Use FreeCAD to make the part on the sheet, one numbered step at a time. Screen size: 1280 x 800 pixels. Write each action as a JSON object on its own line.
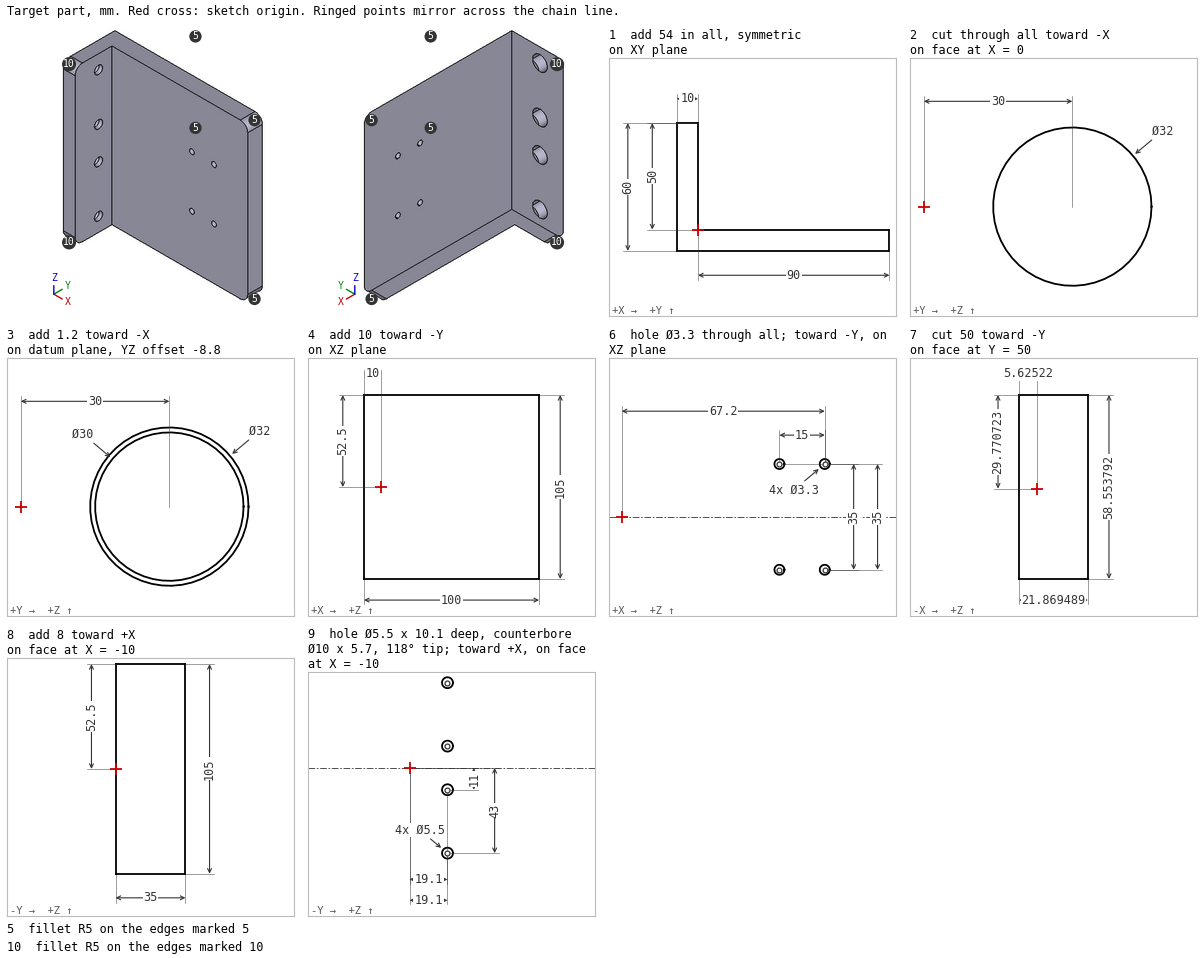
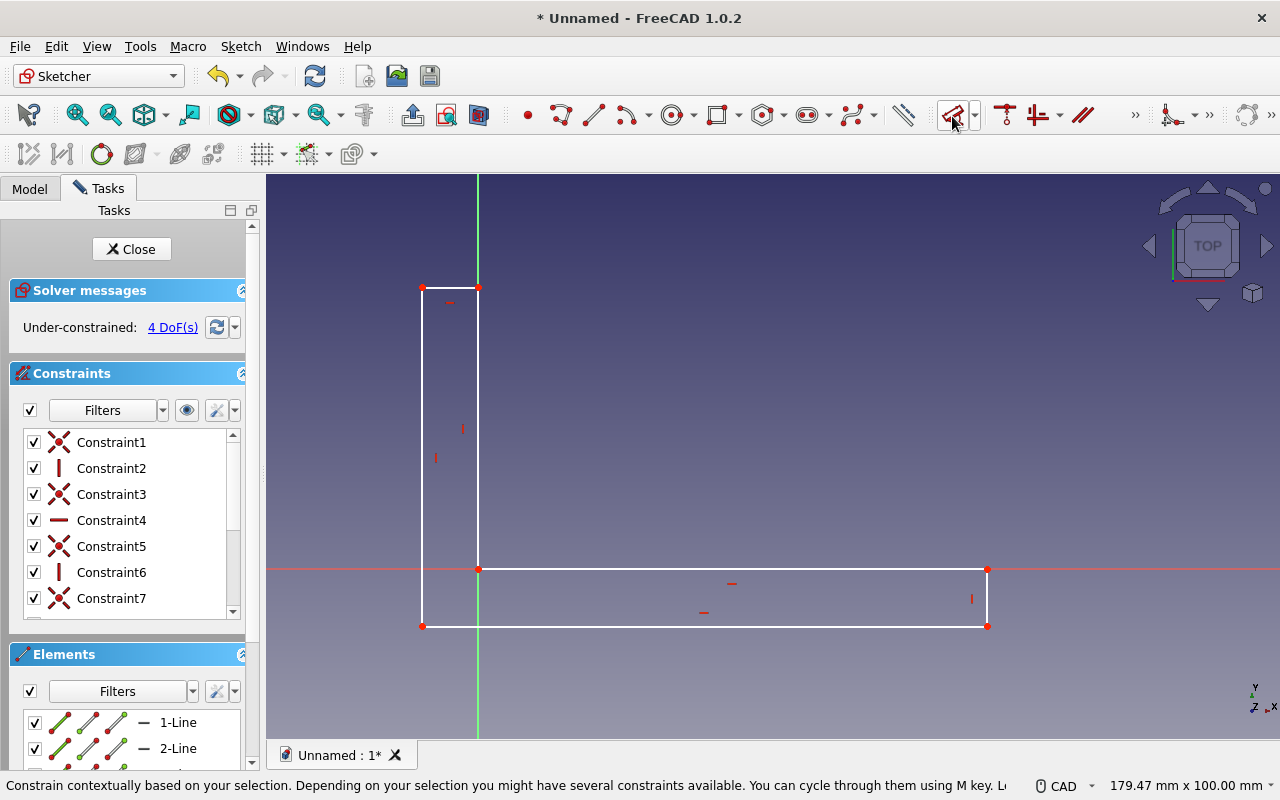
{"action": "left_click", "coordinate": [478, 485]}
{"action": "left_click", "coordinate": [444, 429]}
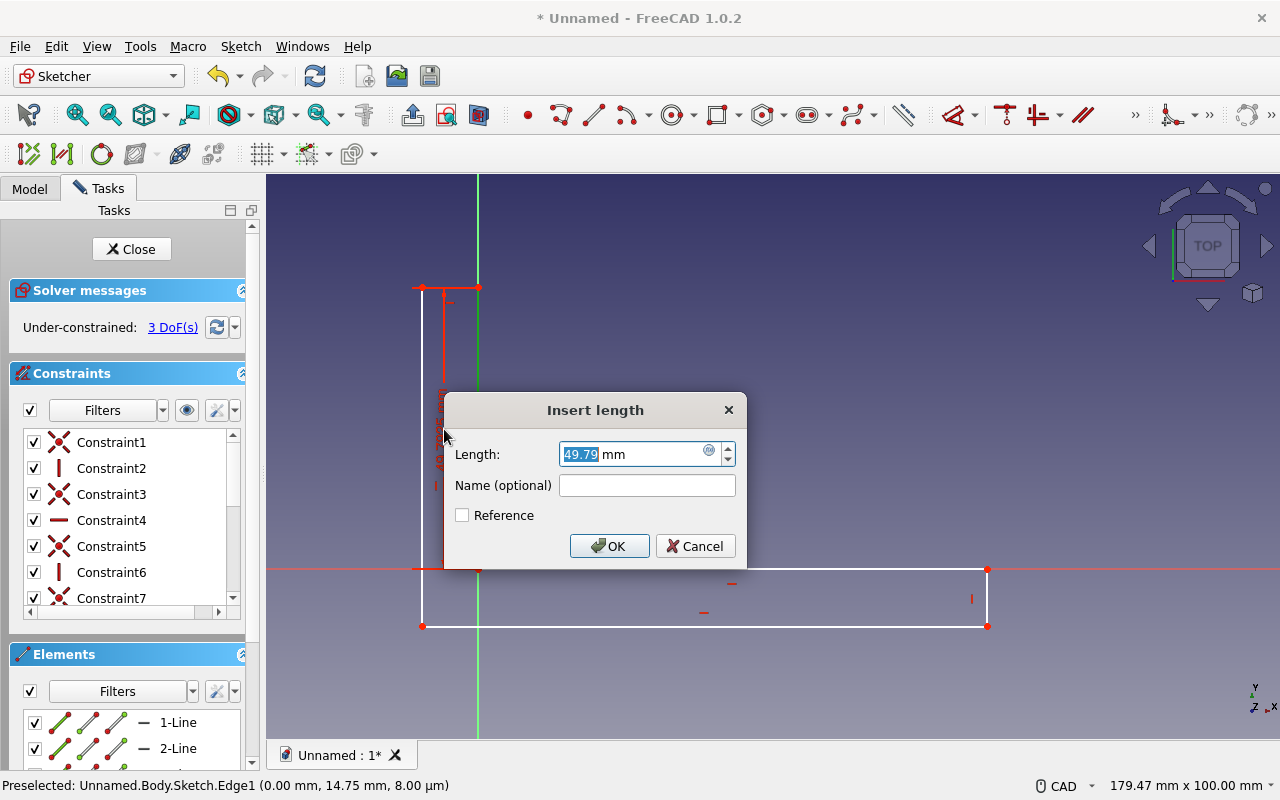
{"action": "type", "text": "50"}
{"action": "key", "text": "Return"}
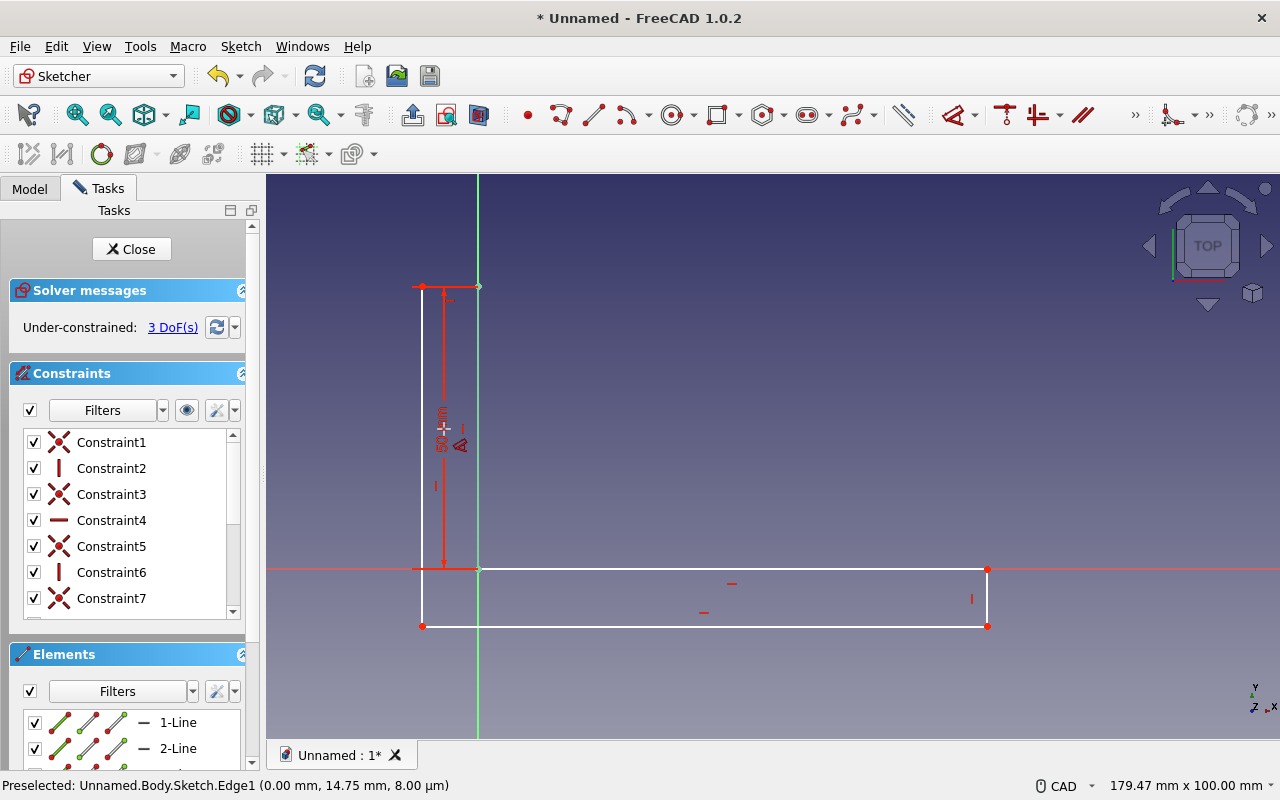
{"action": "left_click", "coordinate": [461, 287]}
{"action": "left_click", "coordinate": [450, 253]}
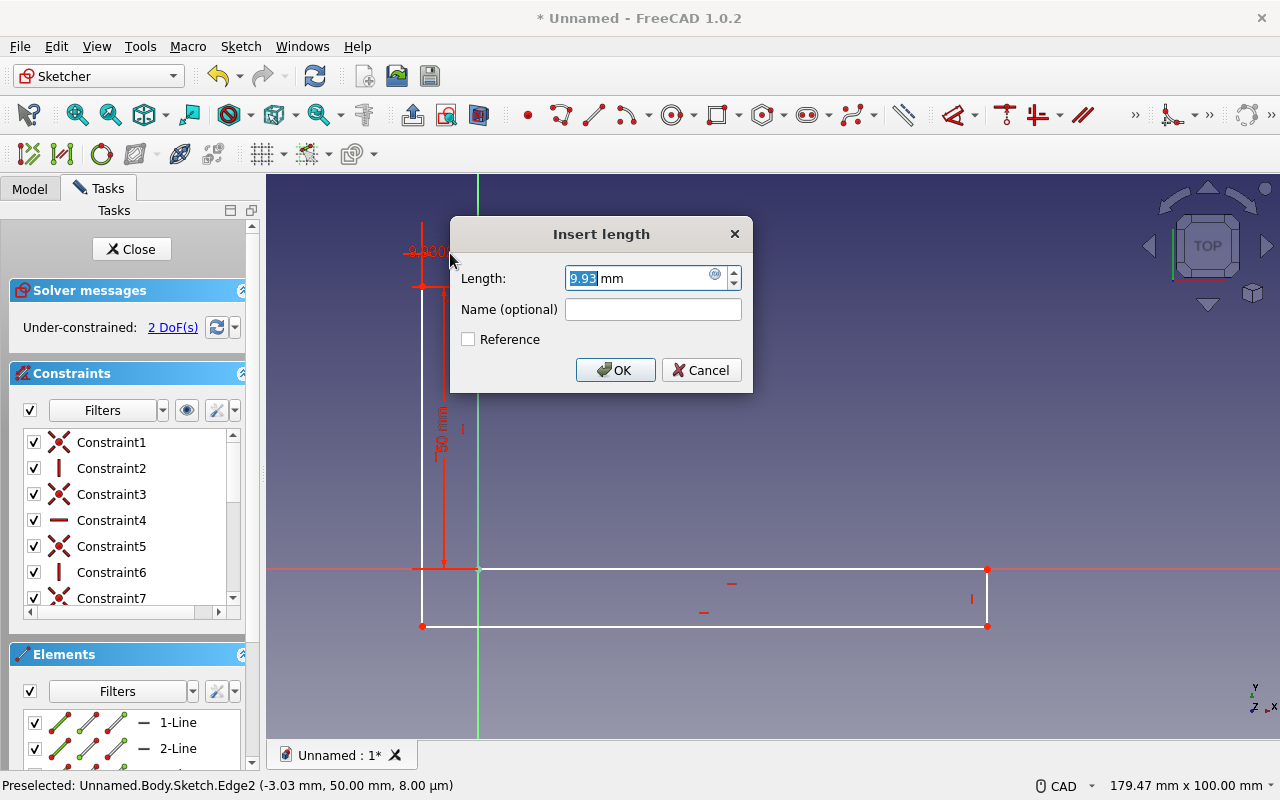
{"action": "type", "text": "10"}
{"action": "key", "text": "Return"}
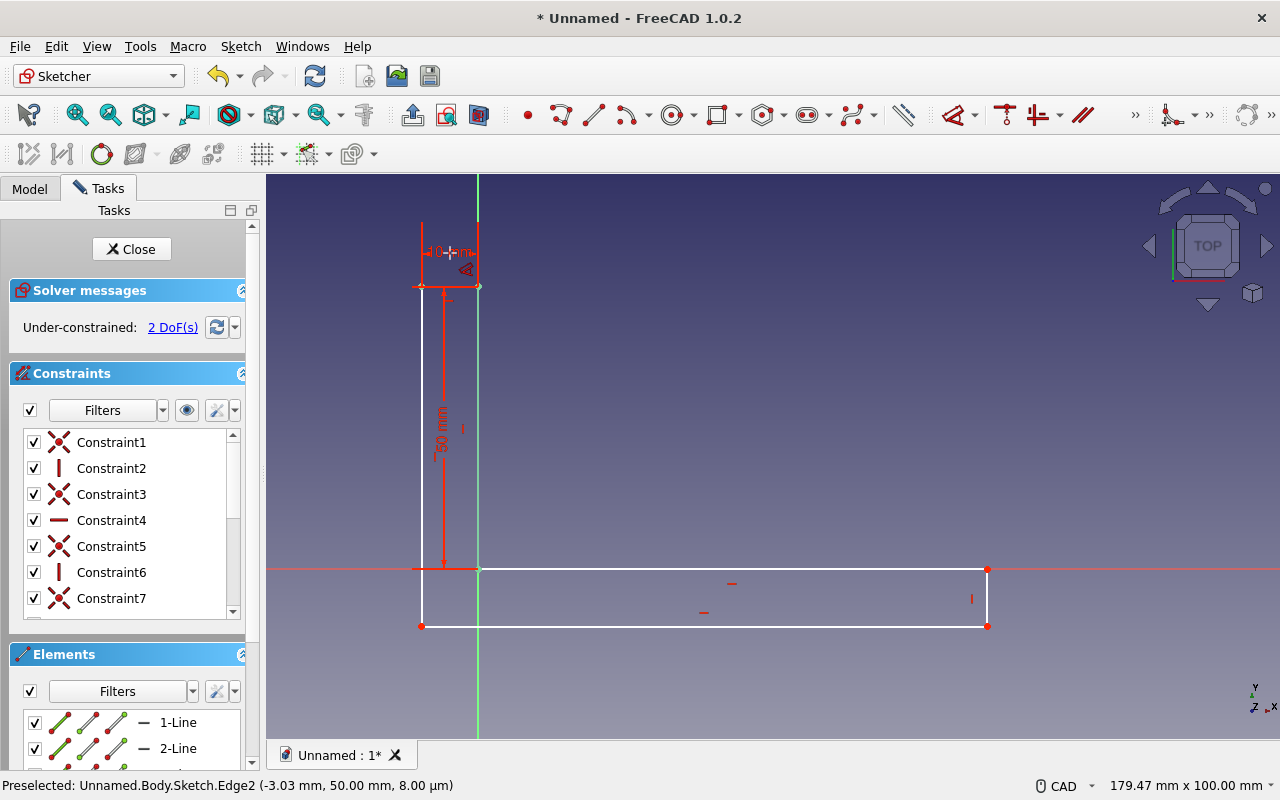
{"action": "left_click", "coordinate": [422, 389]}
{"action": "left_click", "coordinate": [388, 457]}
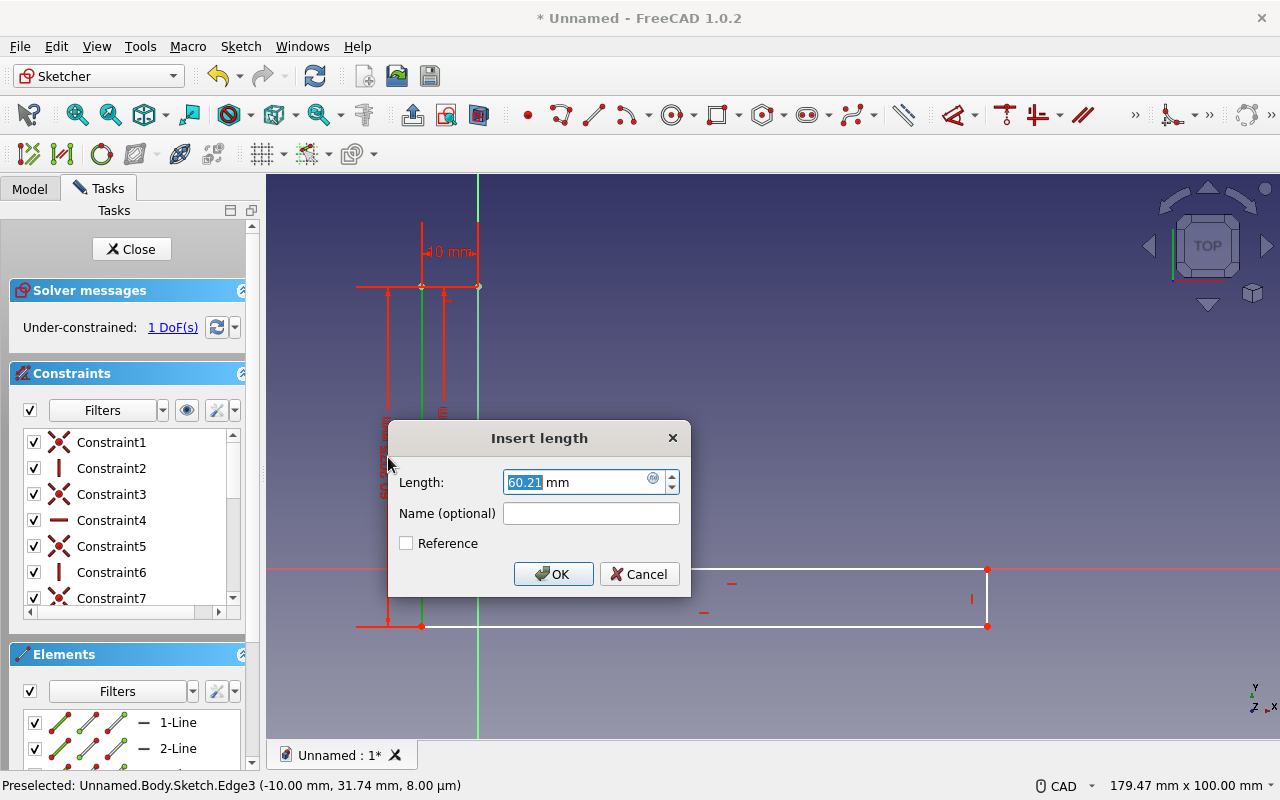
{"action": "type", "text": "60"}
{"action": "key", "text": "Return"}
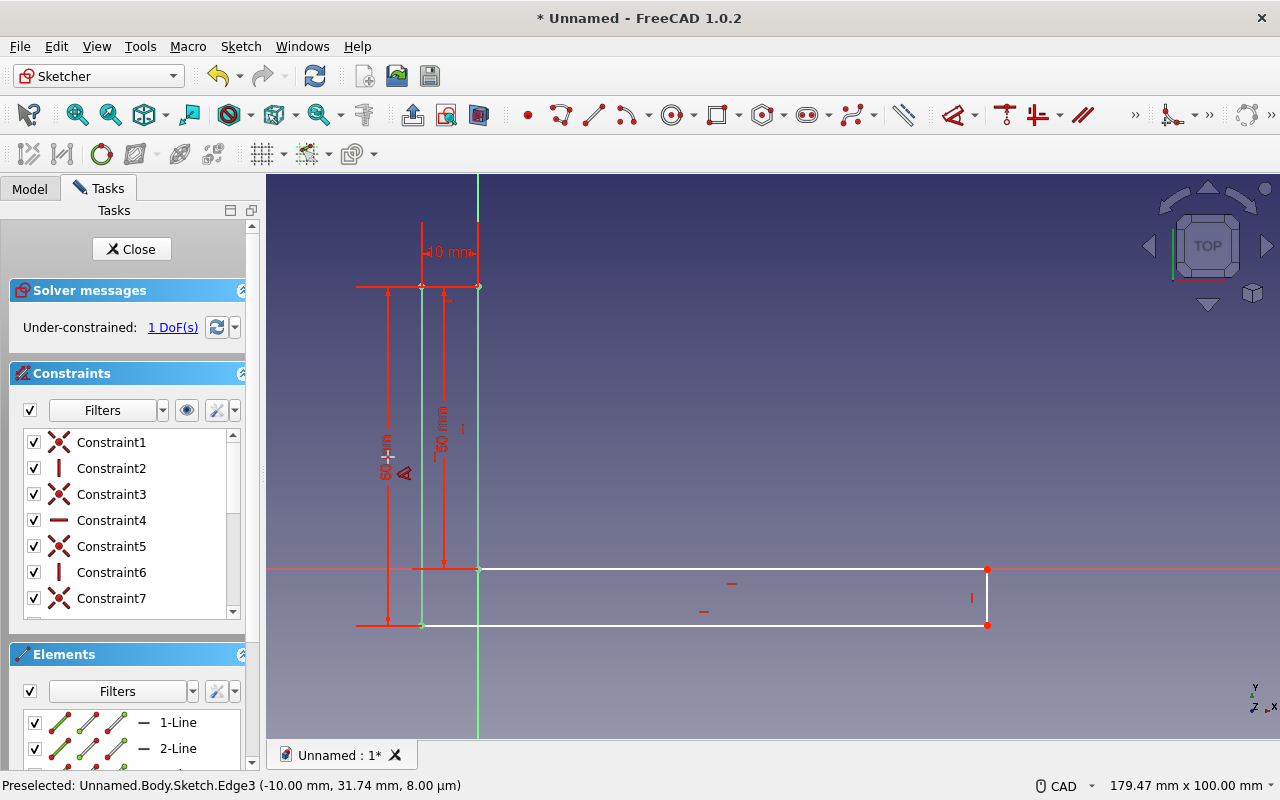
{"action": "left_click", "coordinate": [834, 569]}
{"action": "left_click", "coordinate": [733, 603]}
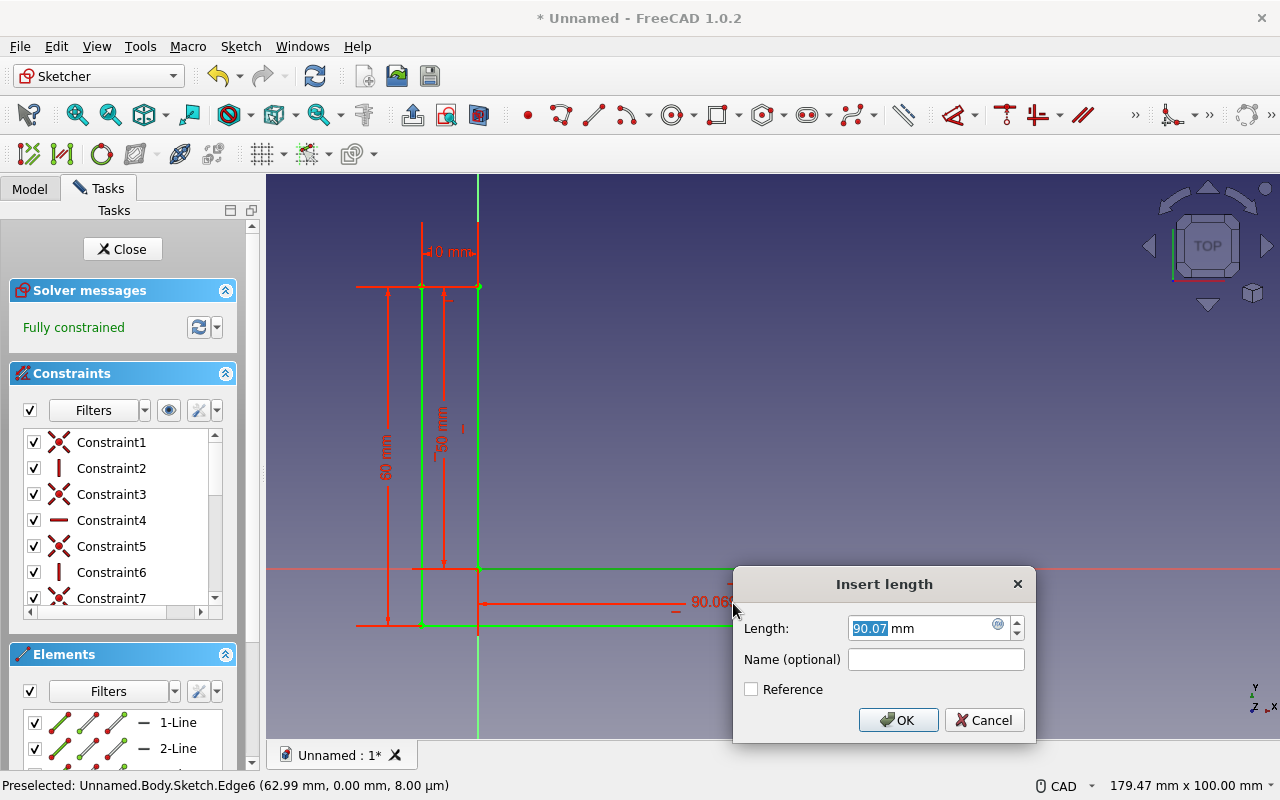
{"action": "type", "text": "90"}
{"action": "key", "text": "Return"}
{"action": "key", "text": "Escape"}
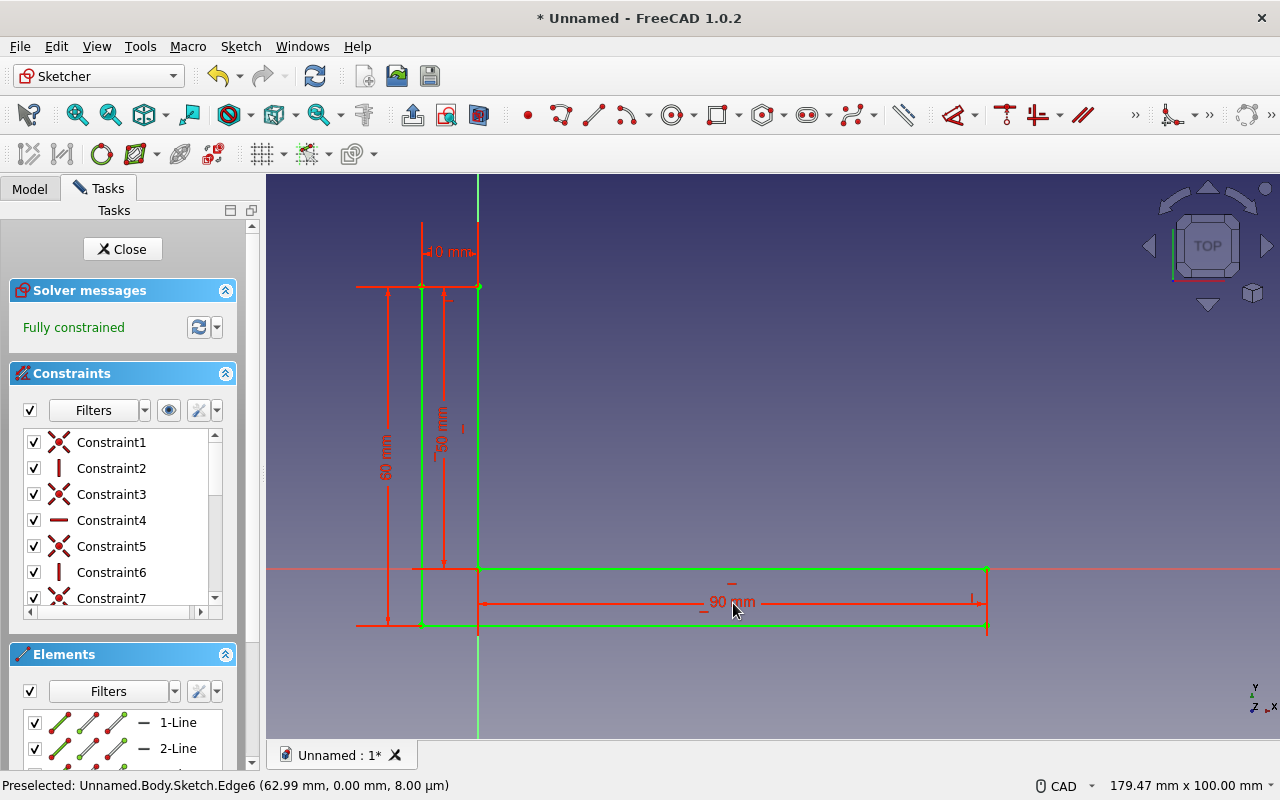
{"action": "left_click", "coordinate": [123, 249]}